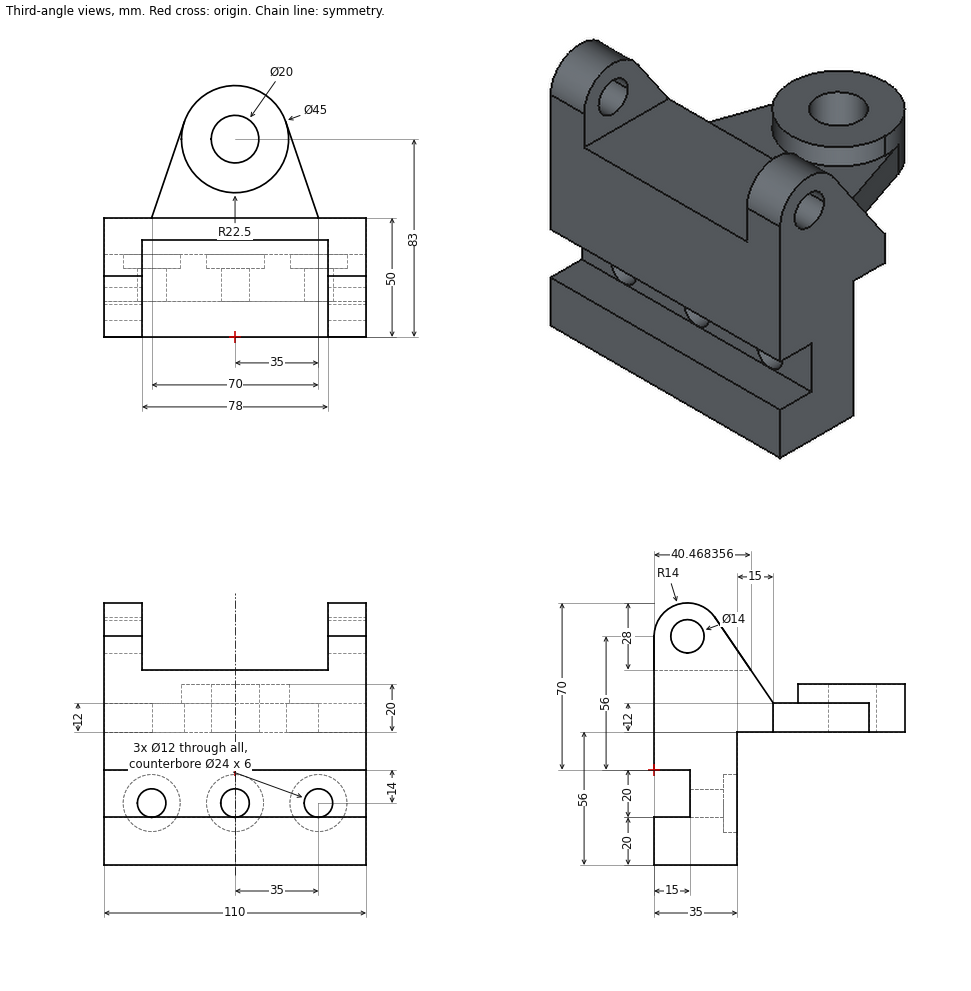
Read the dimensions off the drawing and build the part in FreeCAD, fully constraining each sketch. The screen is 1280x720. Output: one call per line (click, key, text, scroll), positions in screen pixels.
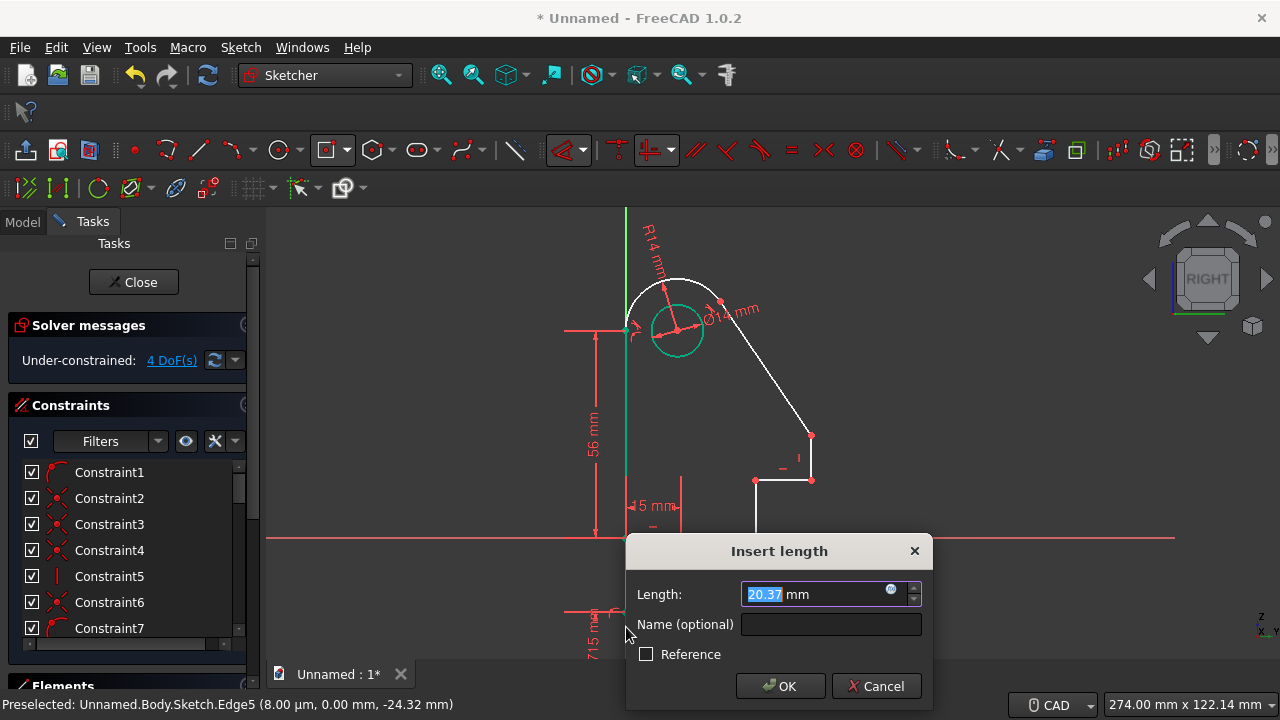
text(20)
key(Return)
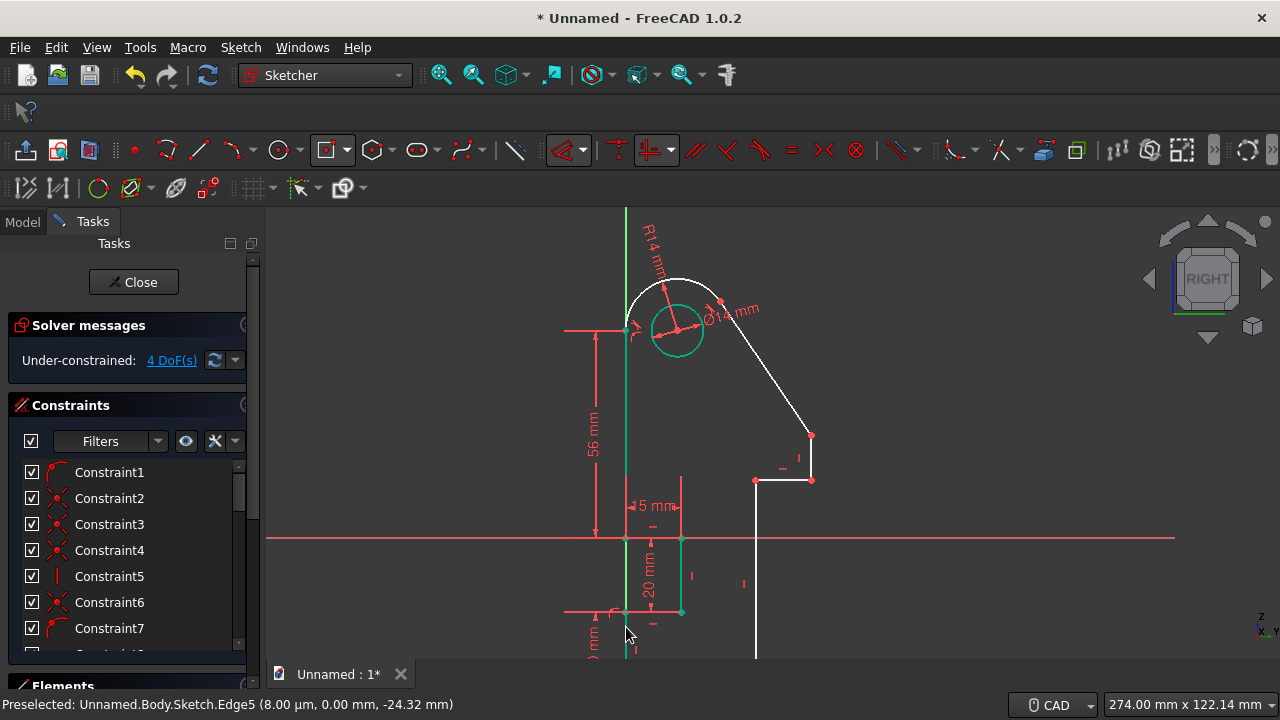
scroll(677, 330, down, 2)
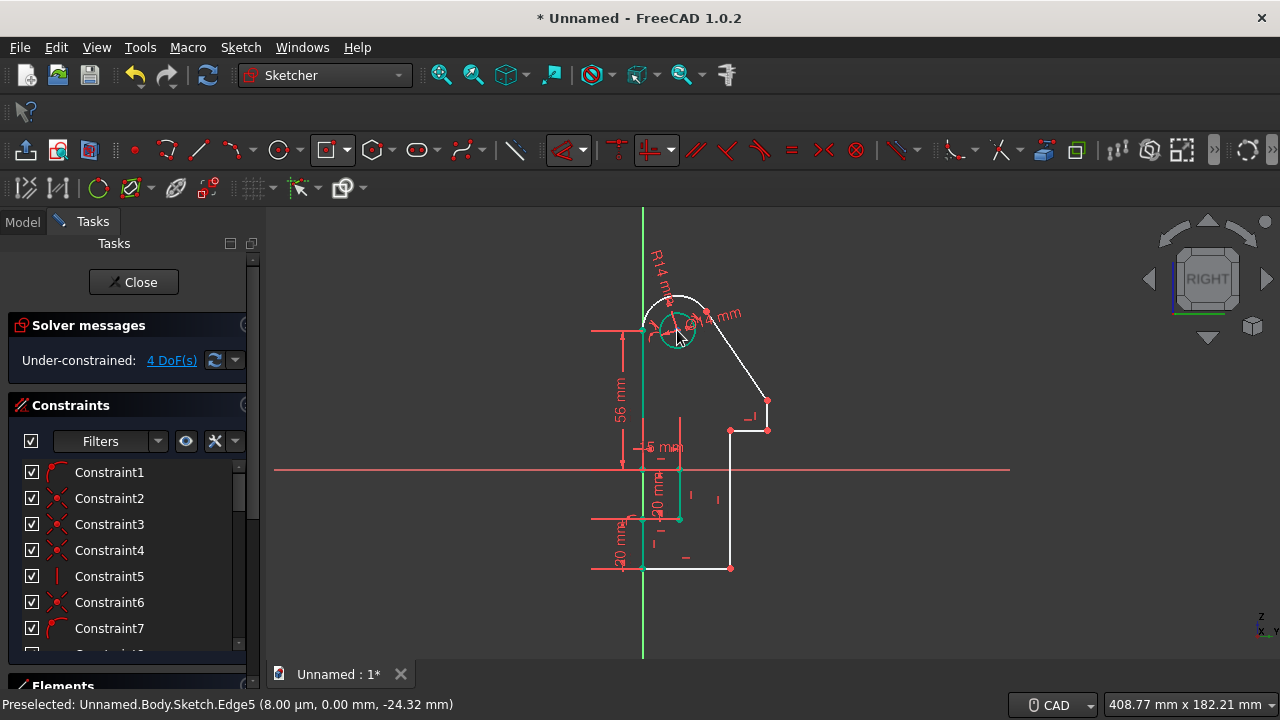
click(669, 569)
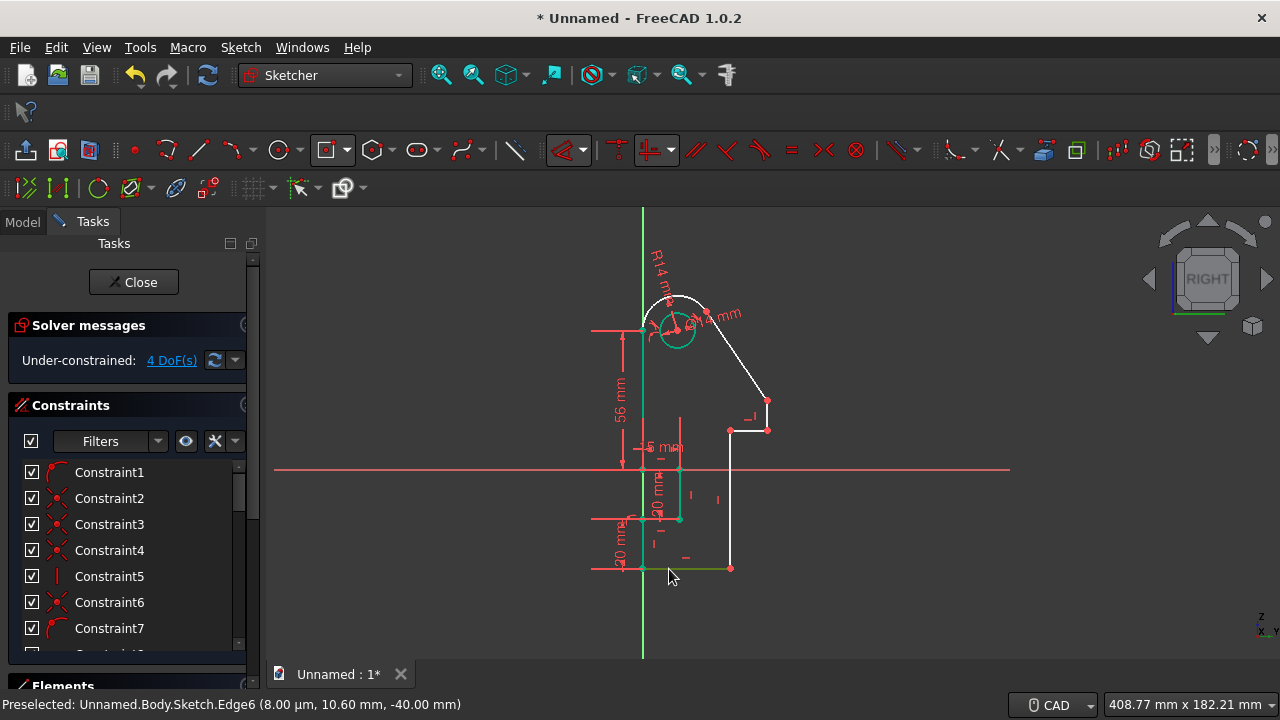
click(586, 150)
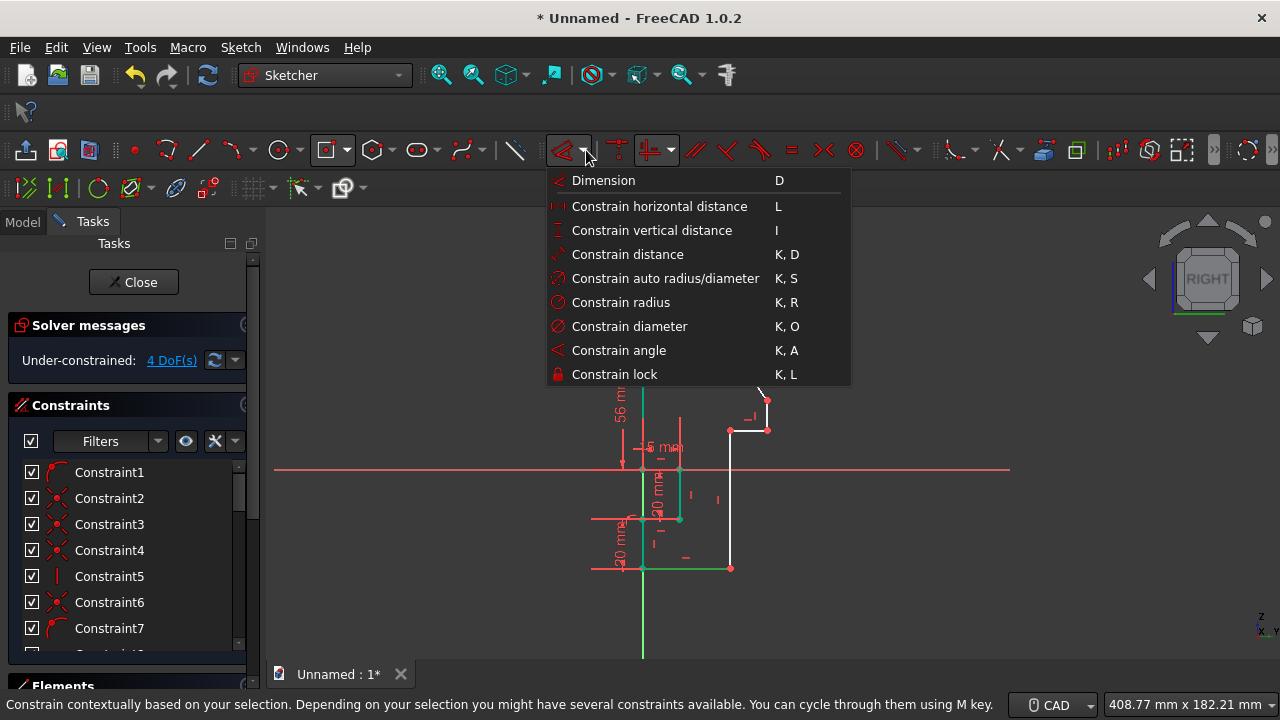
click(699, 206)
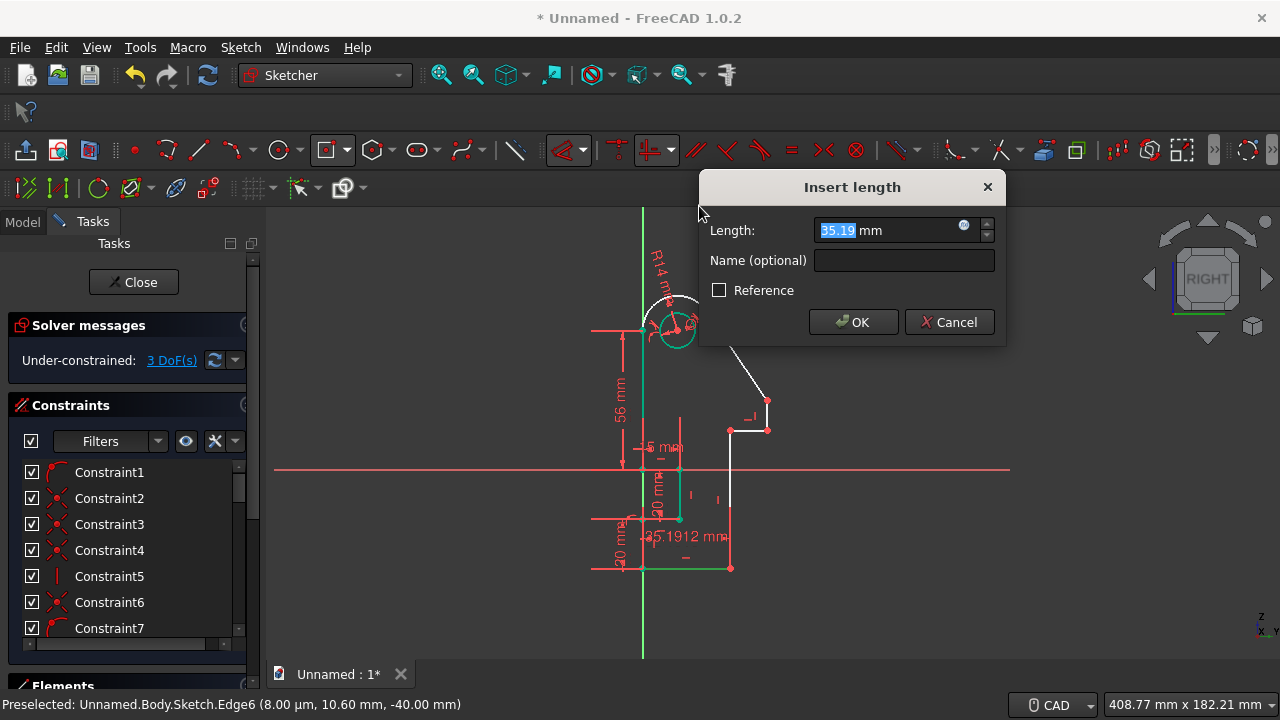
text(35)
key(Return)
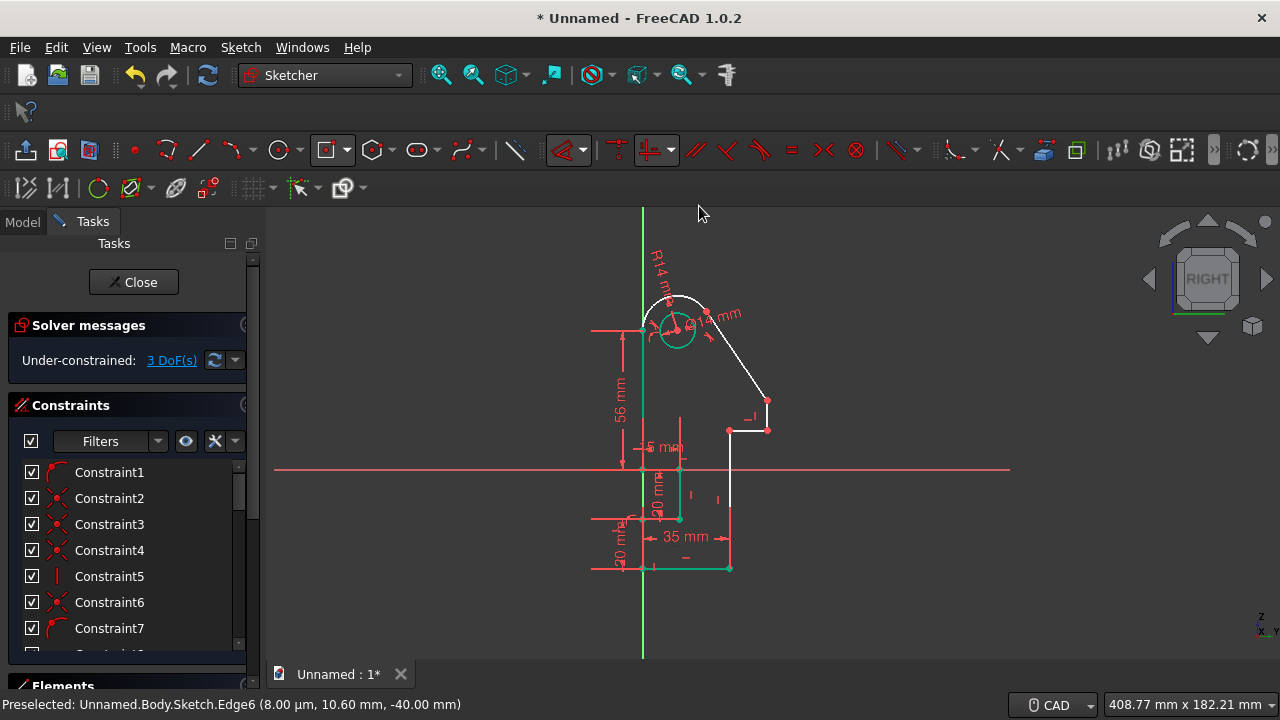
click(730, 527)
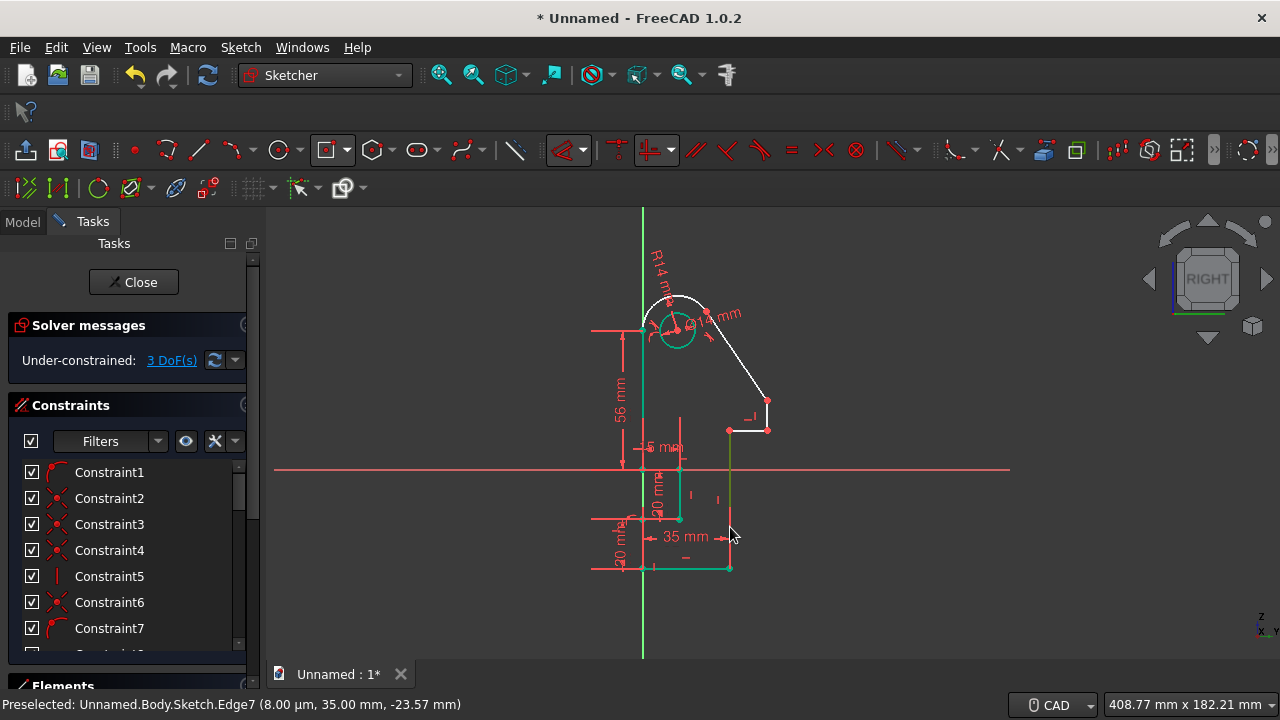
click(586, 150)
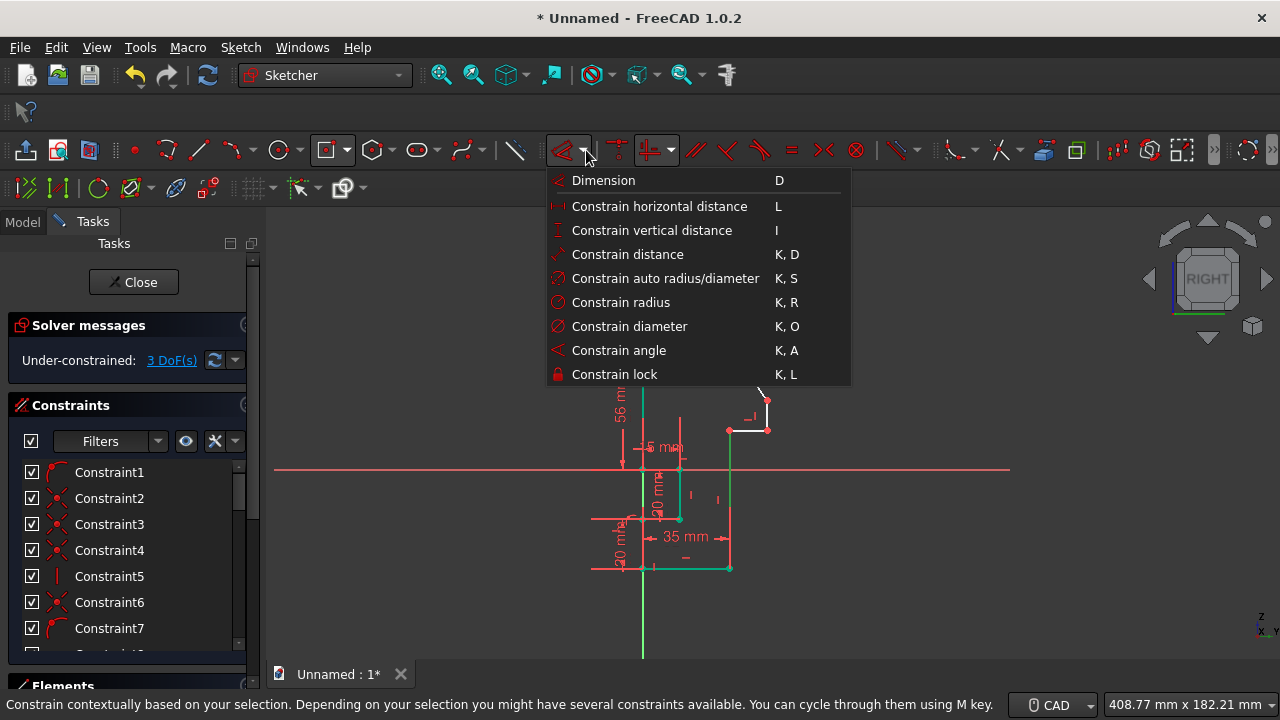
click(699, 230)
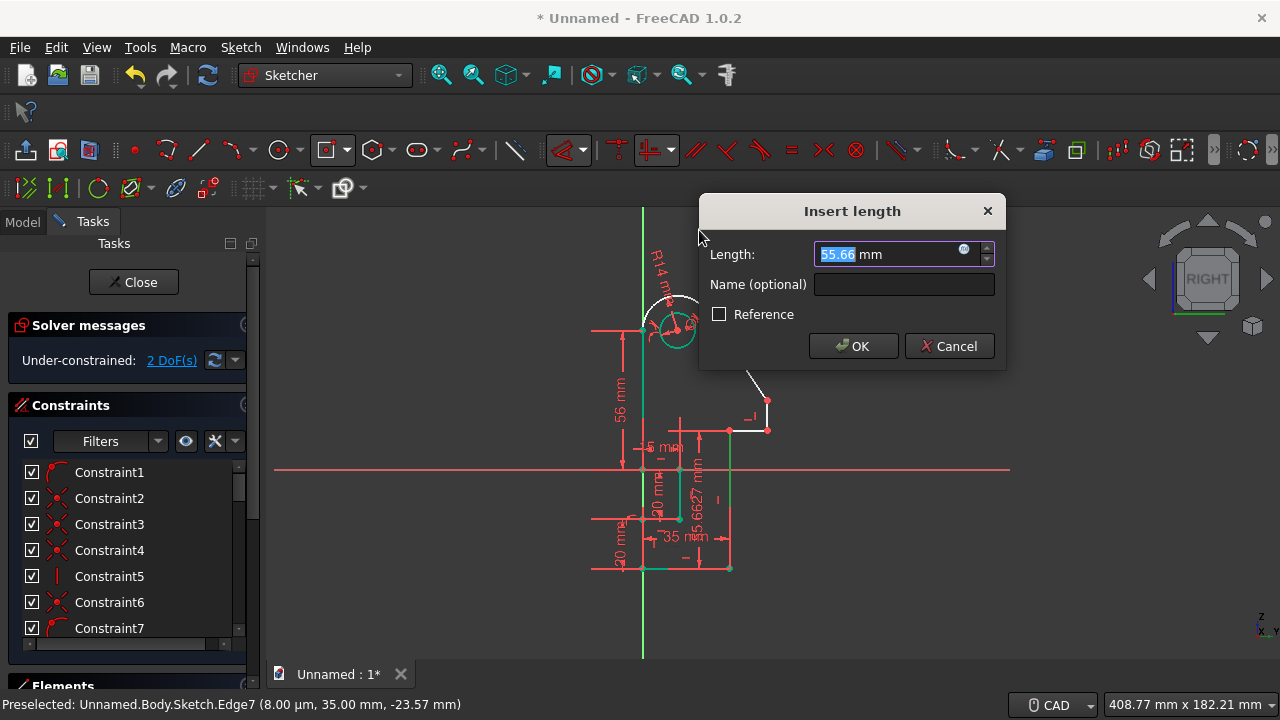
text(56)
key(Return)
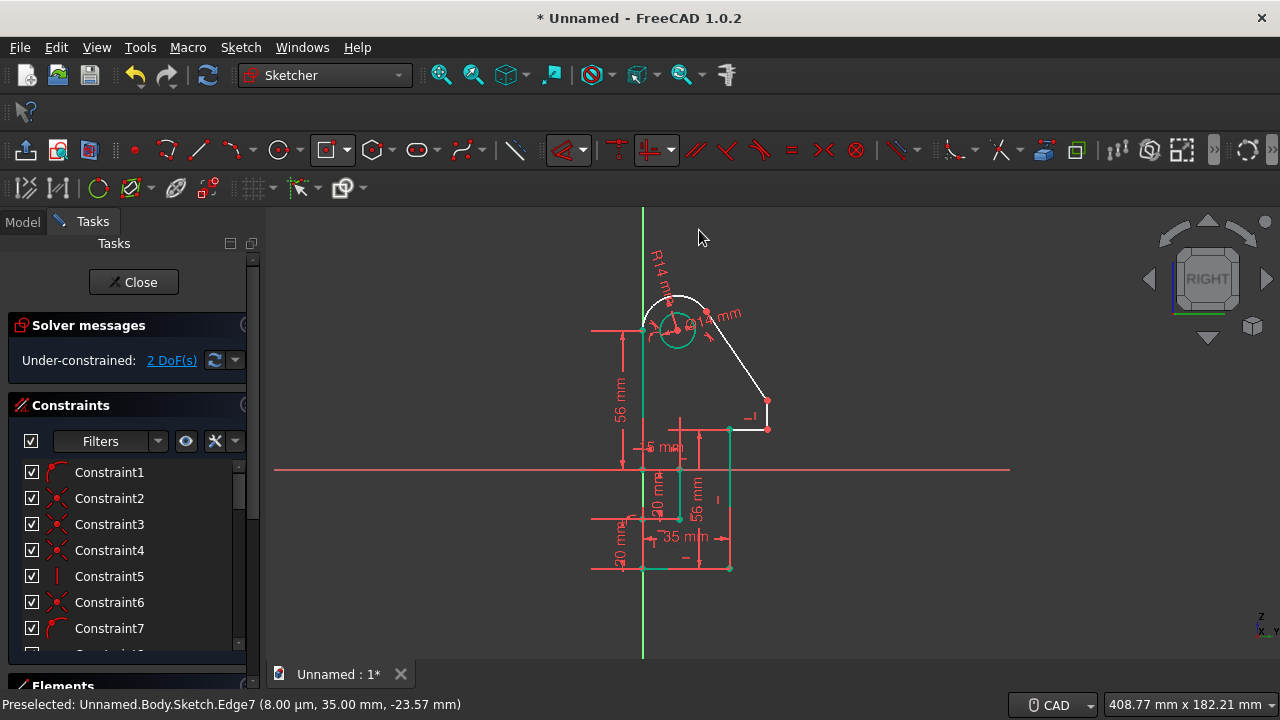
scroll(741, 430, up, 2)